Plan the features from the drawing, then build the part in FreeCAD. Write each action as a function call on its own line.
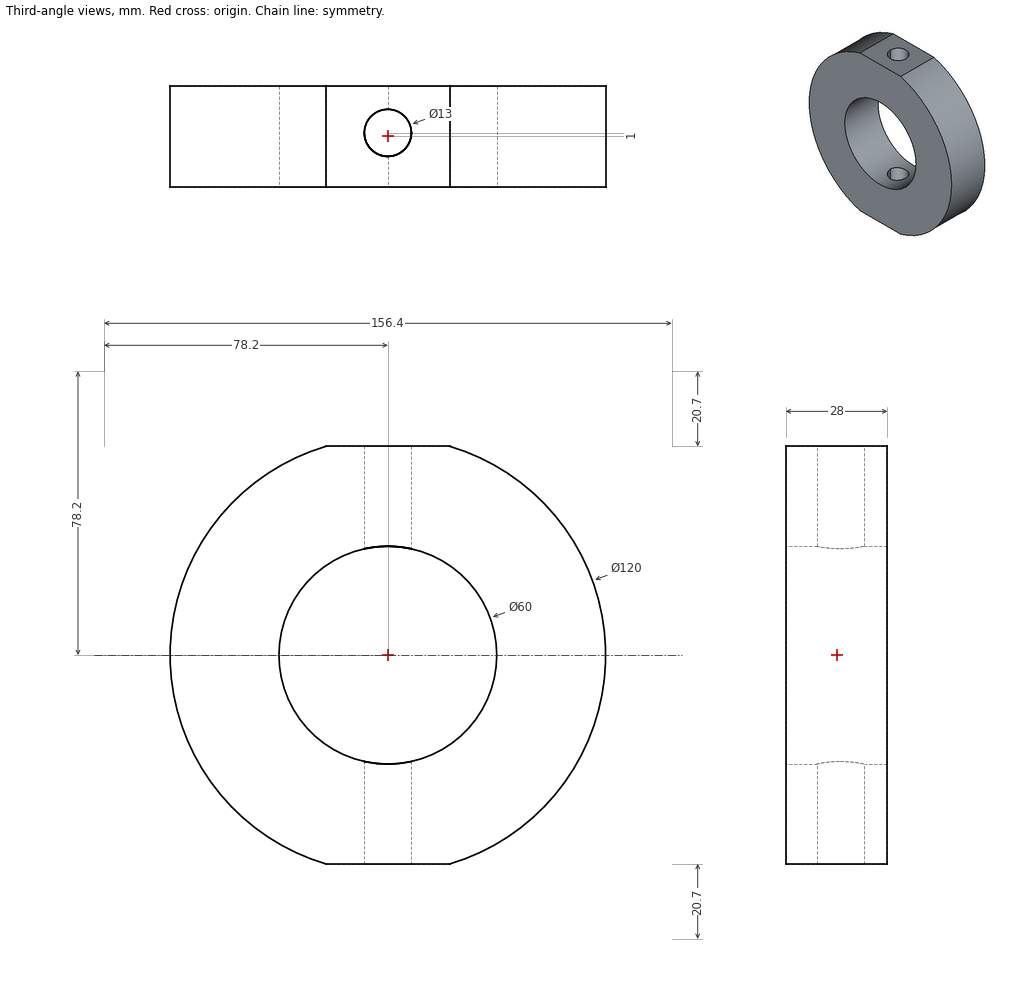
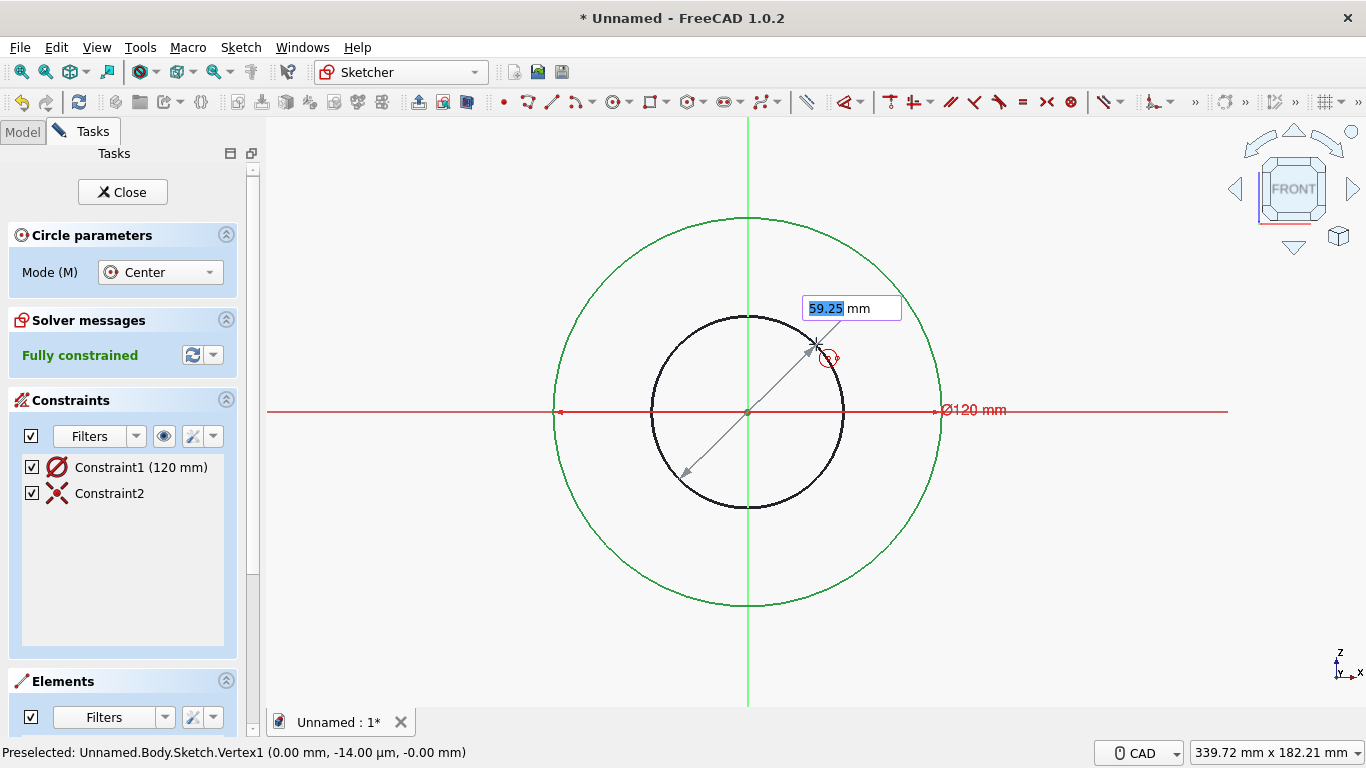
text(60)
key(Return)
key(Escape)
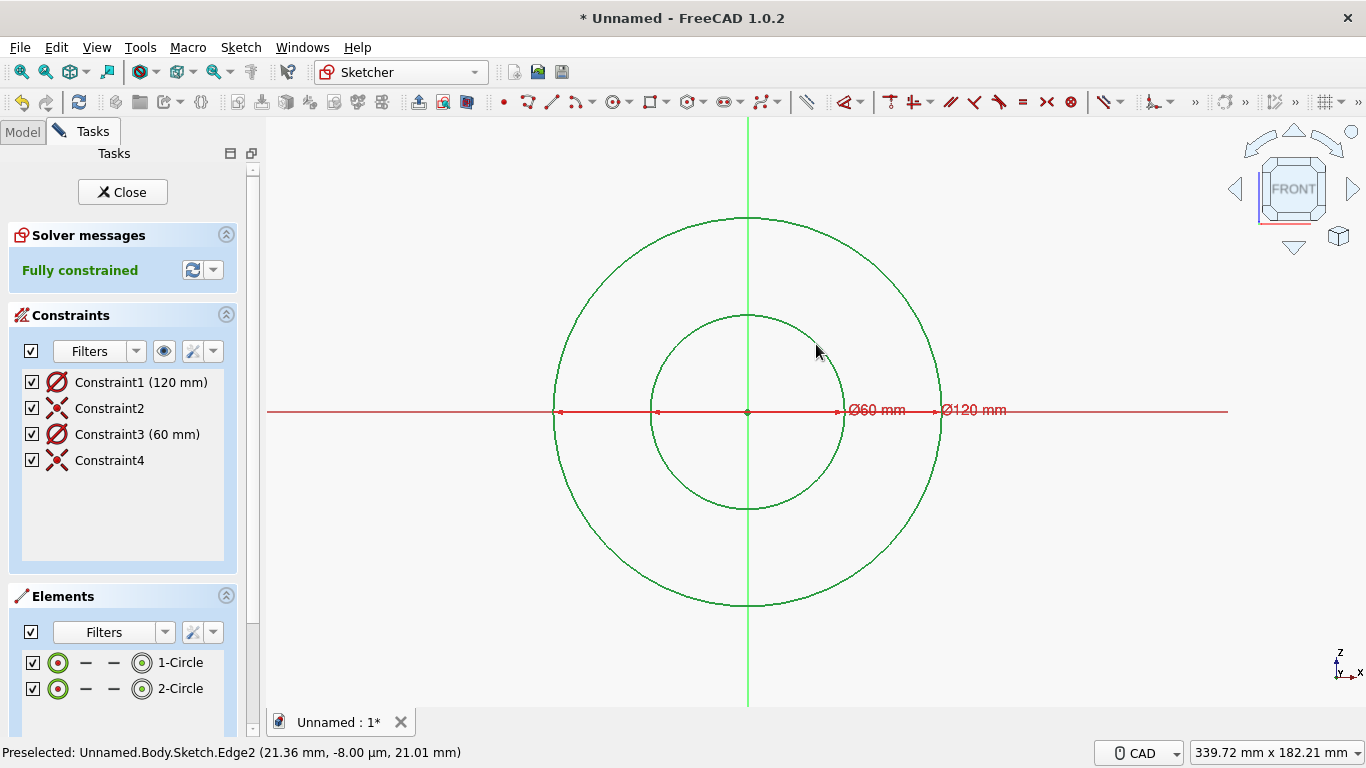
click(123, 192)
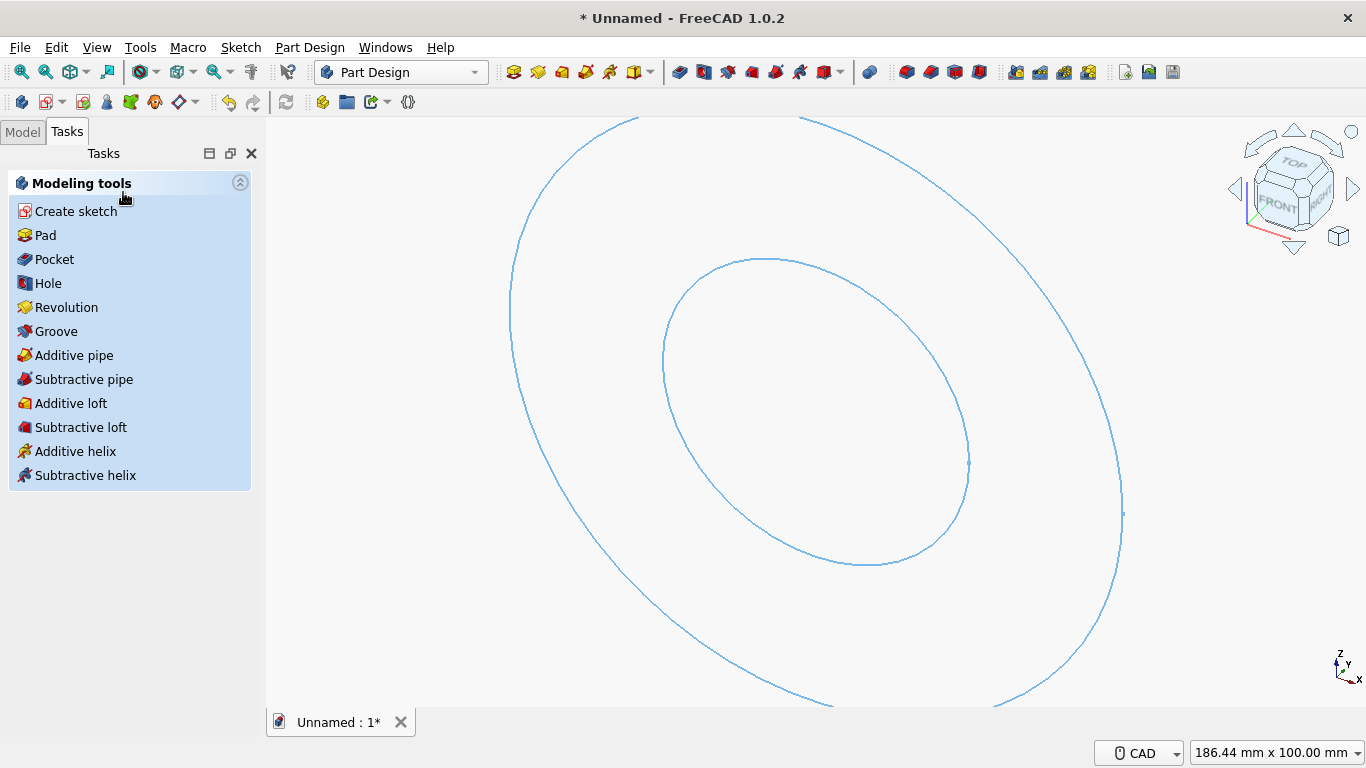
click(514, 72)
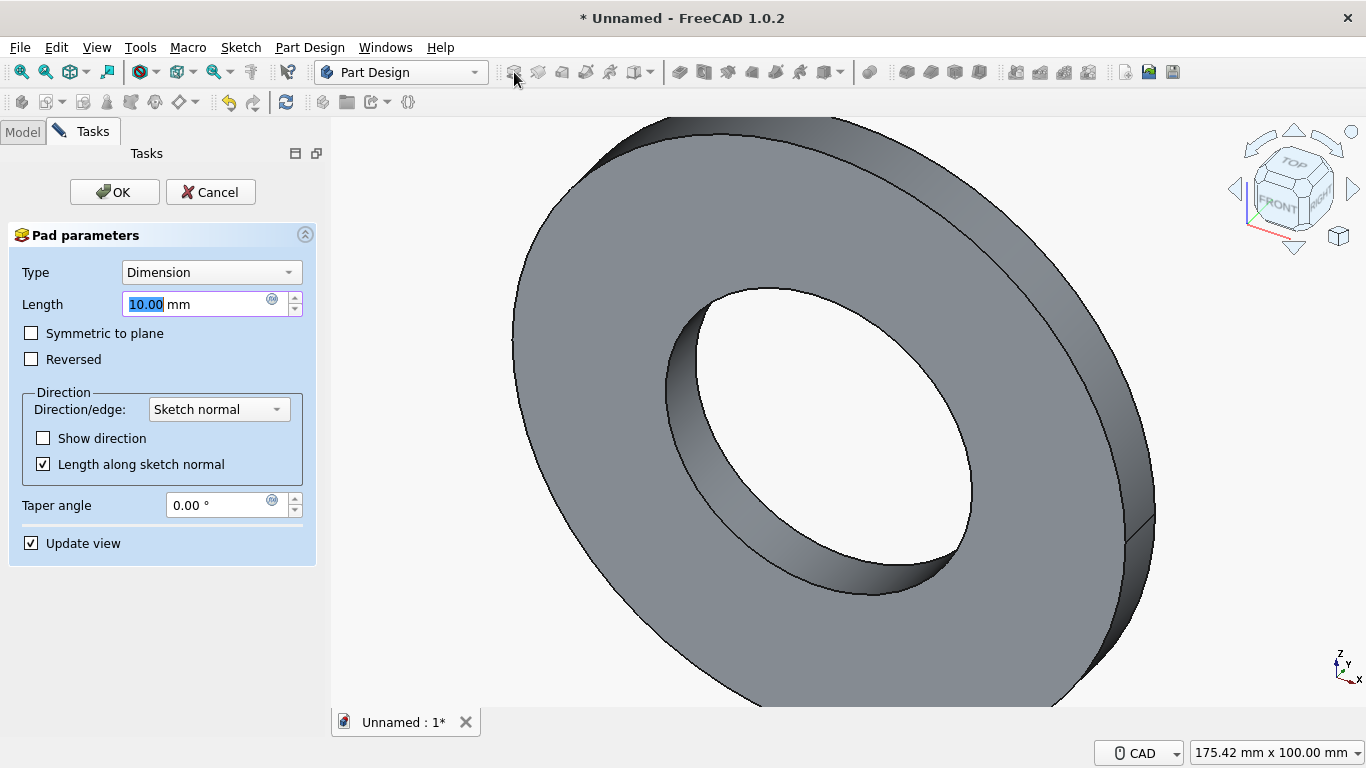
text(28)
key(Tab)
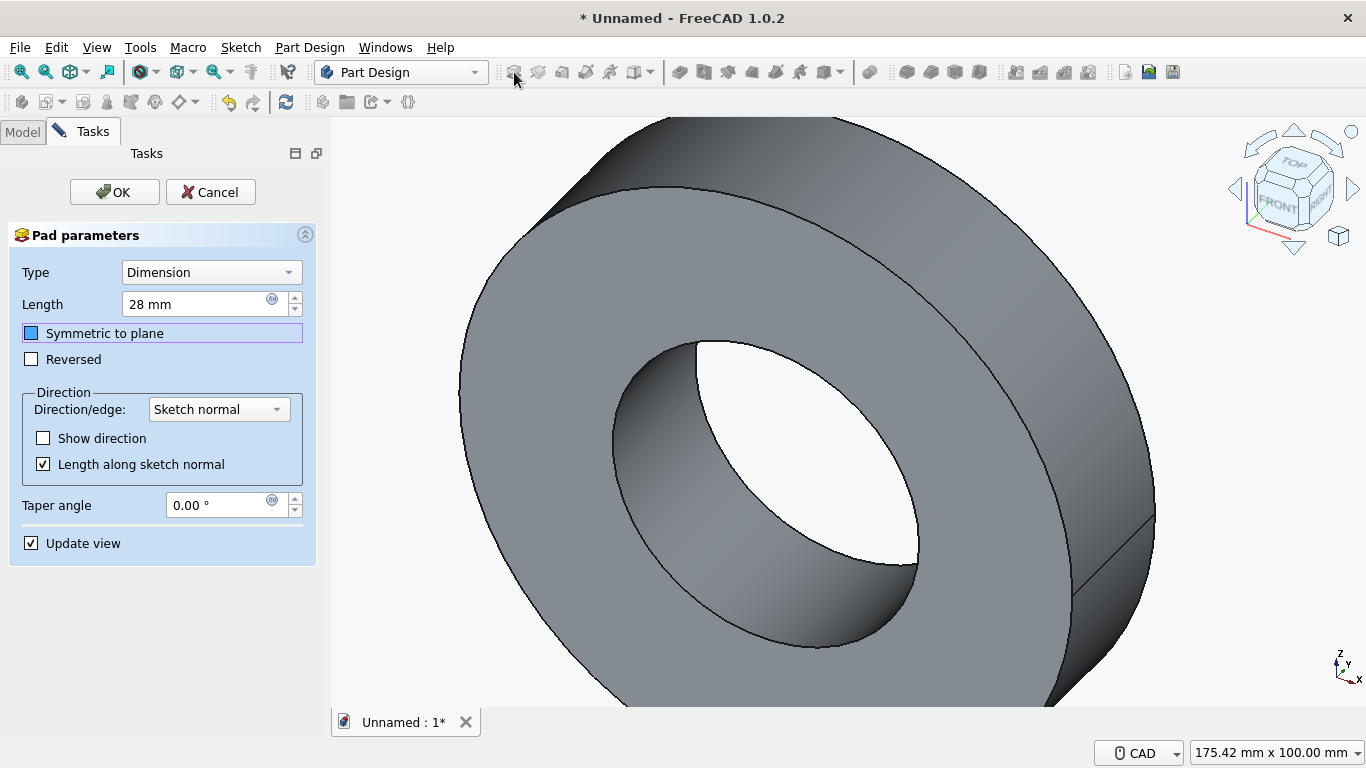
click(30, 333)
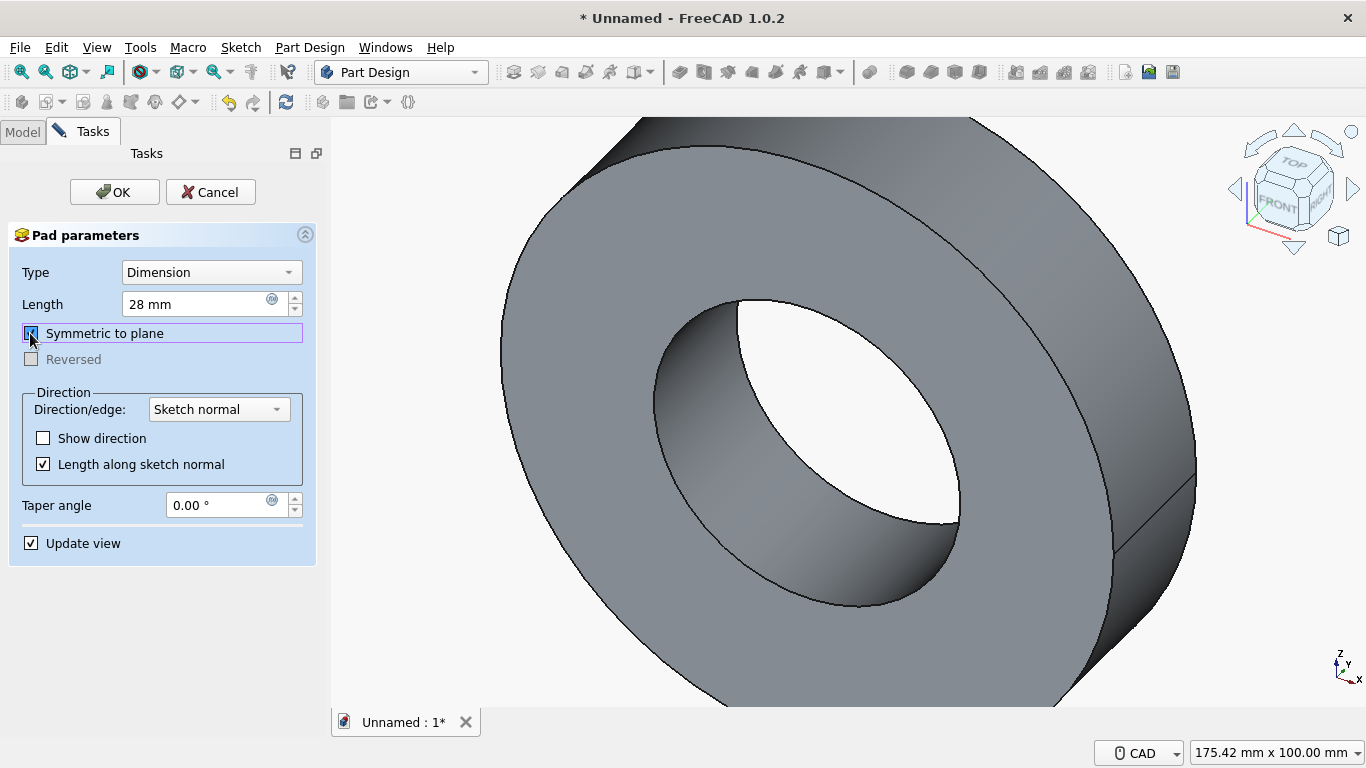
click(115, 192)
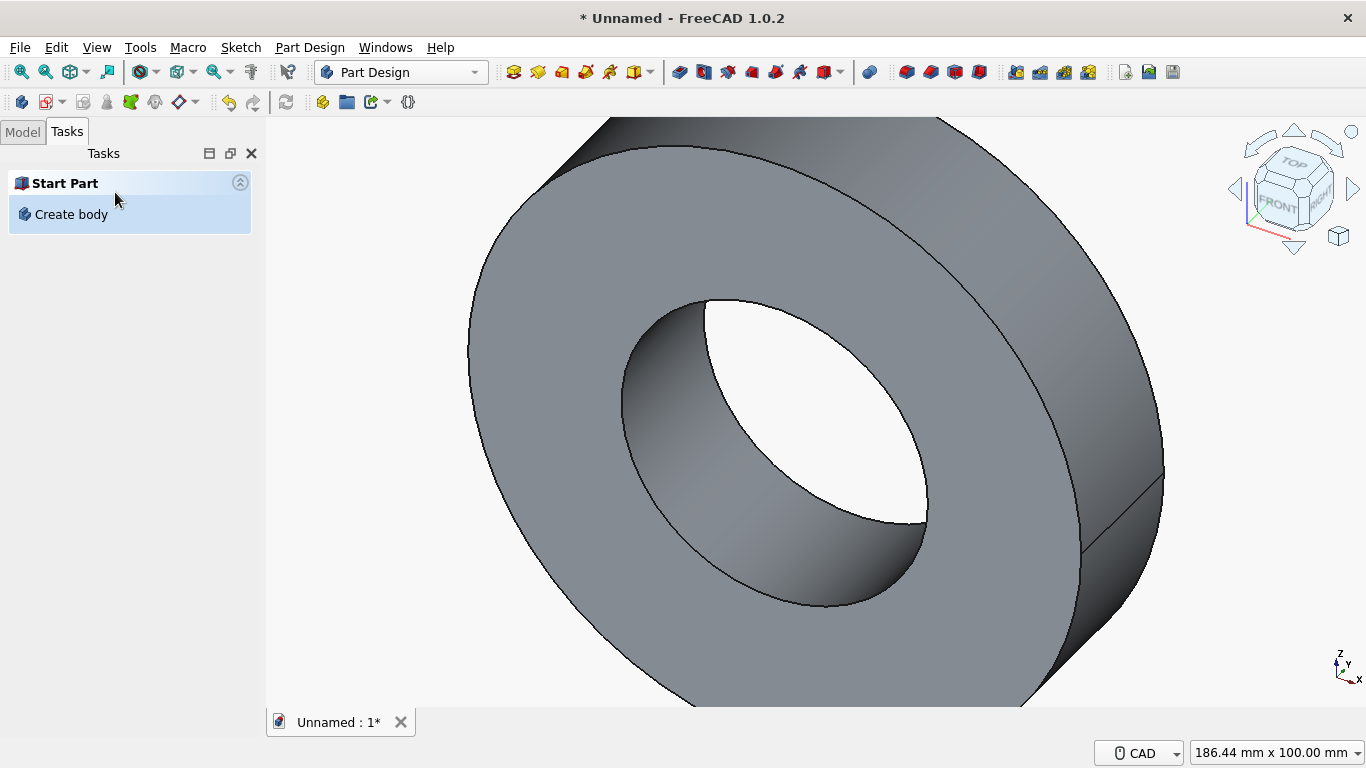
key(v)
key(f)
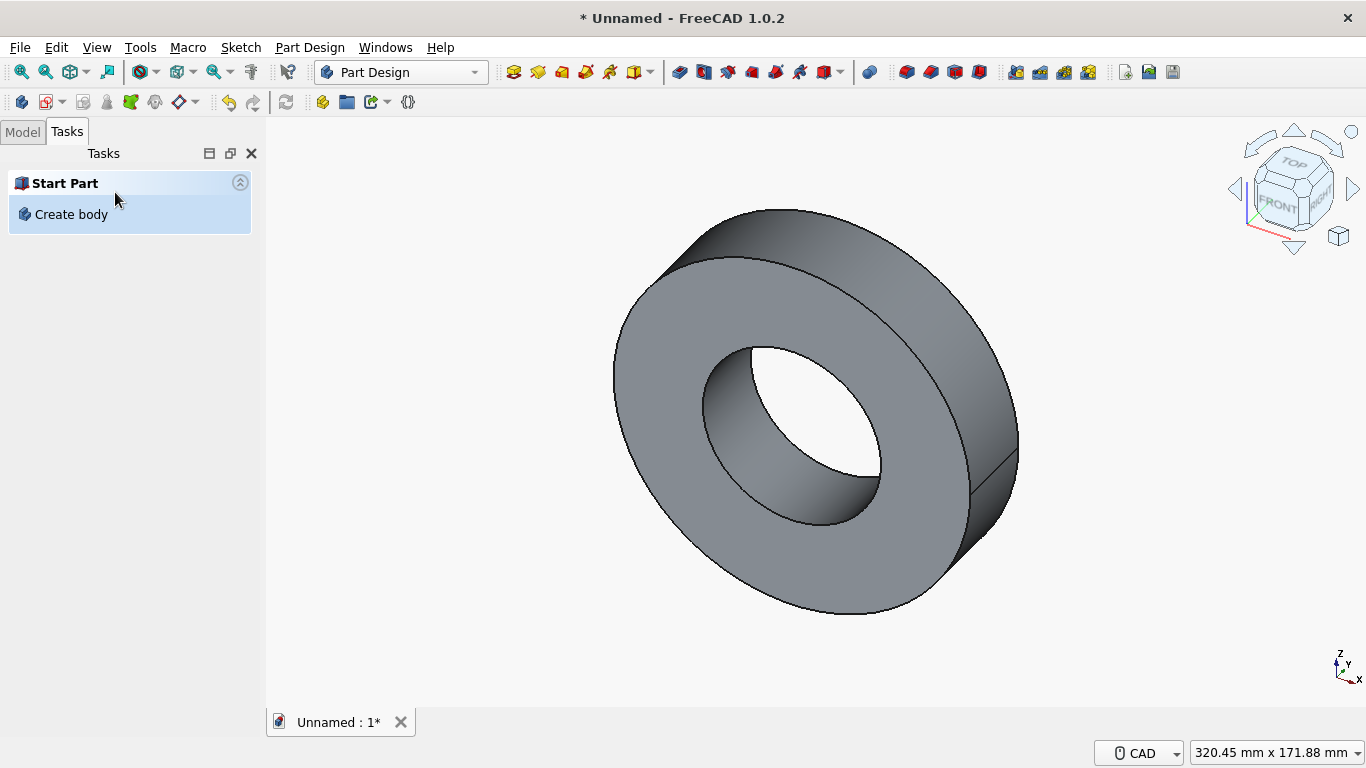
click(46, 102)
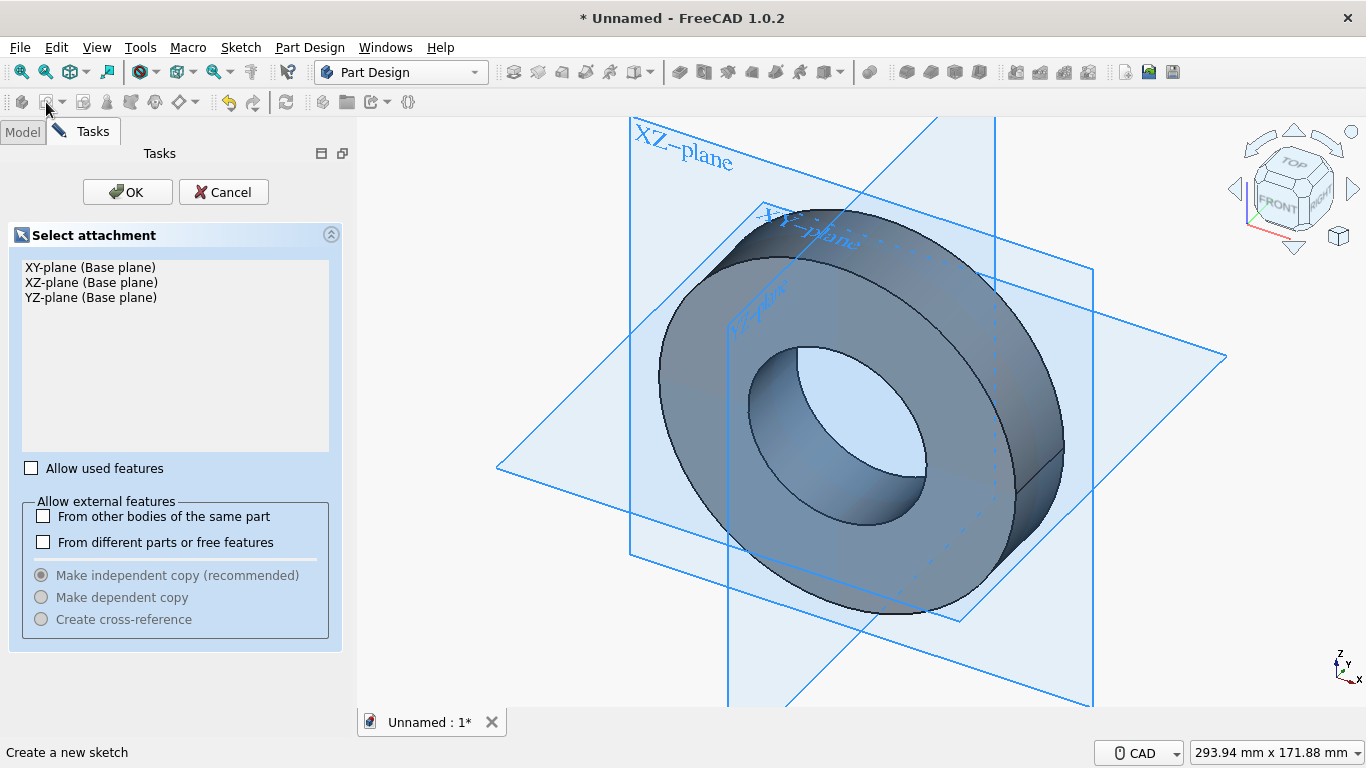
click(82, 282)